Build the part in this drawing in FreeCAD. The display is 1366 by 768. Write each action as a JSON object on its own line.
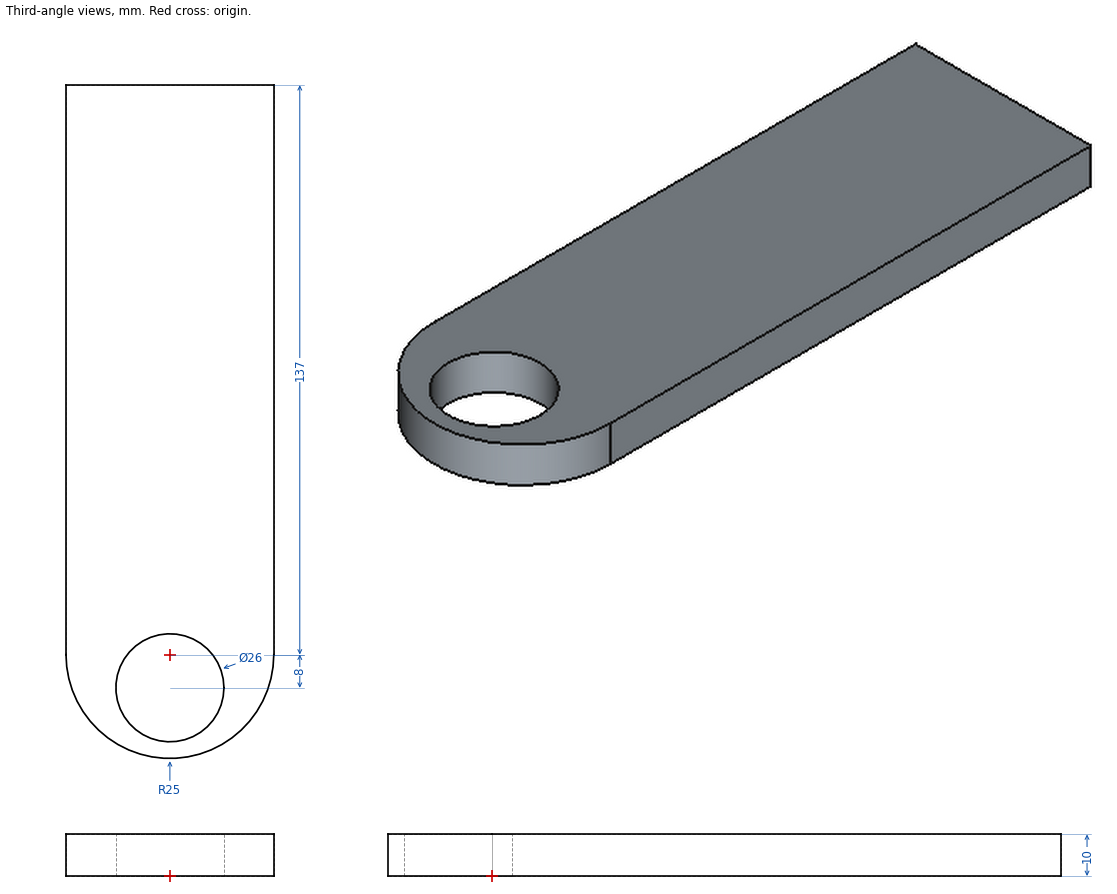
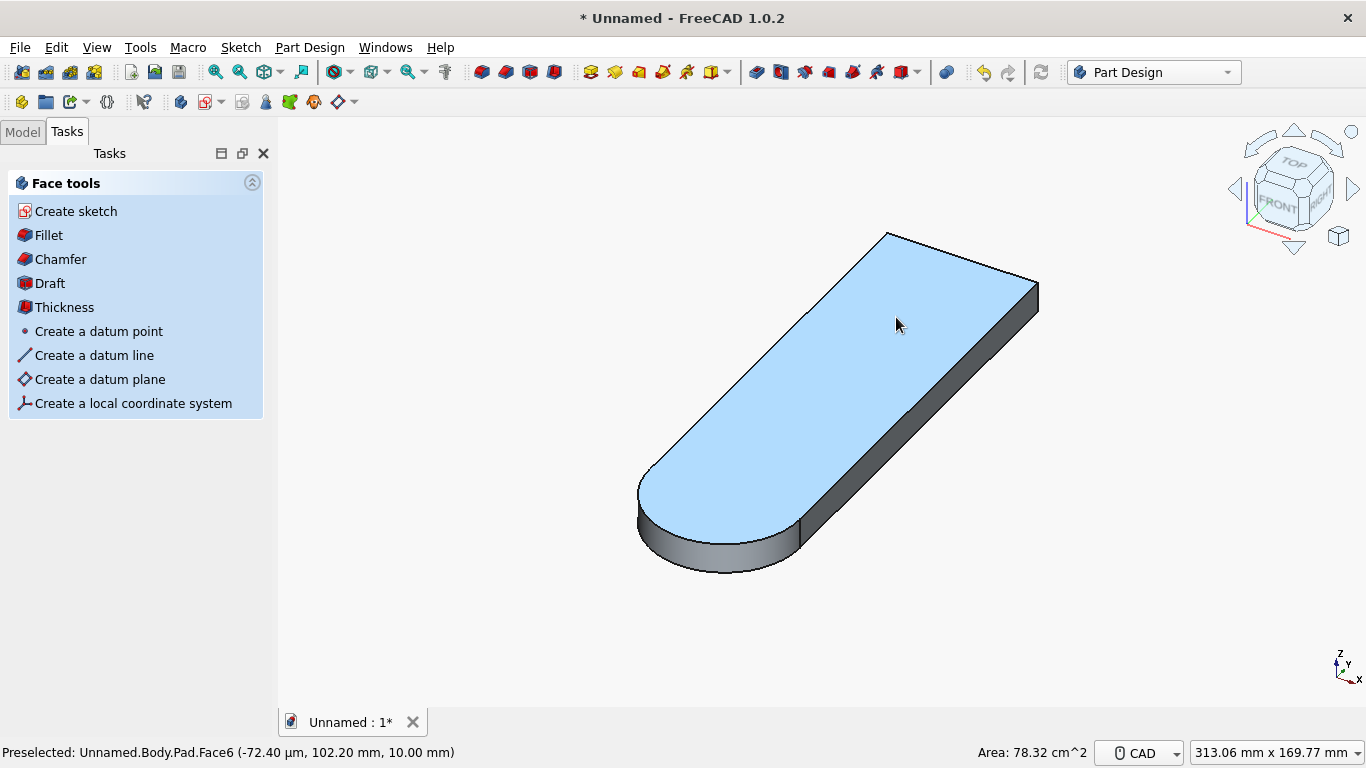
{"action": "left_click", "coordinate": [206, 102]}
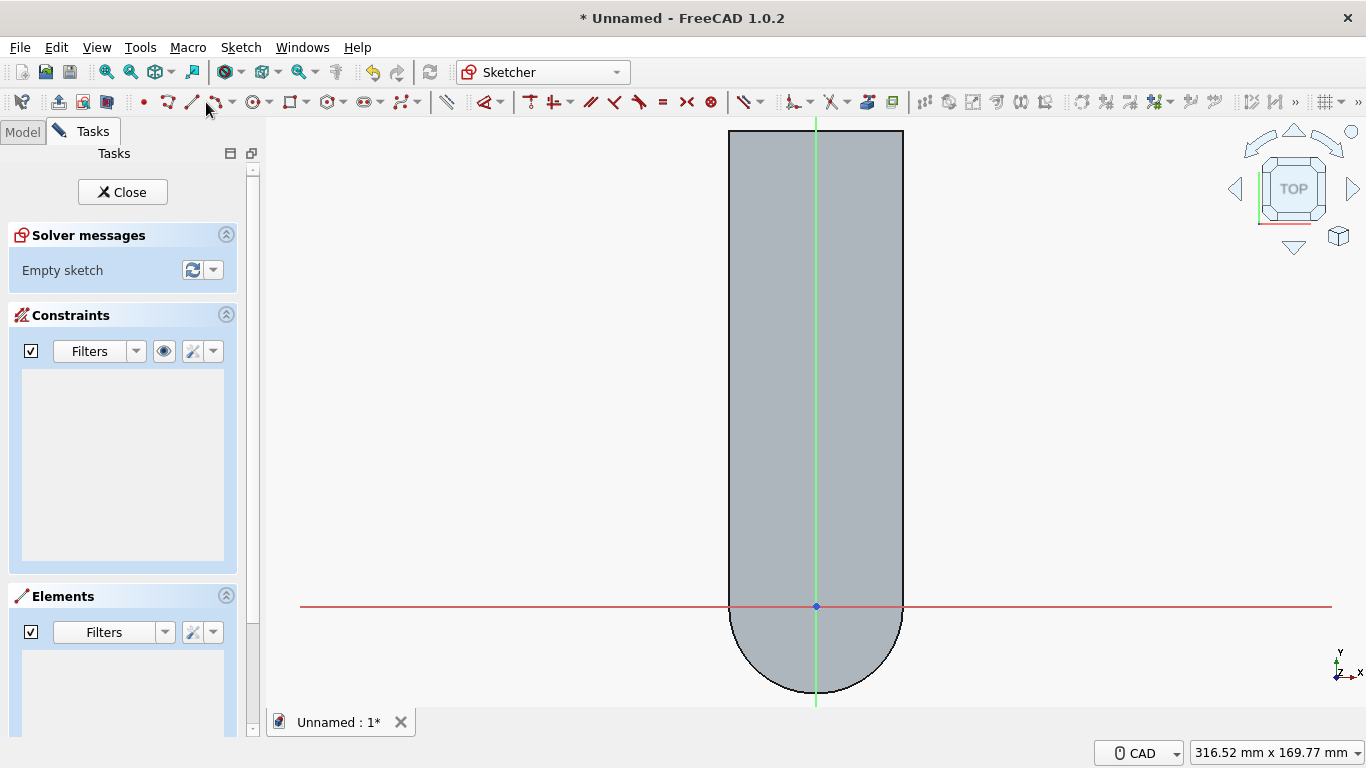
{"action": "scroll", "coordinate": [748, 412], "scroll_direction": "down", "scroll_amount": 5}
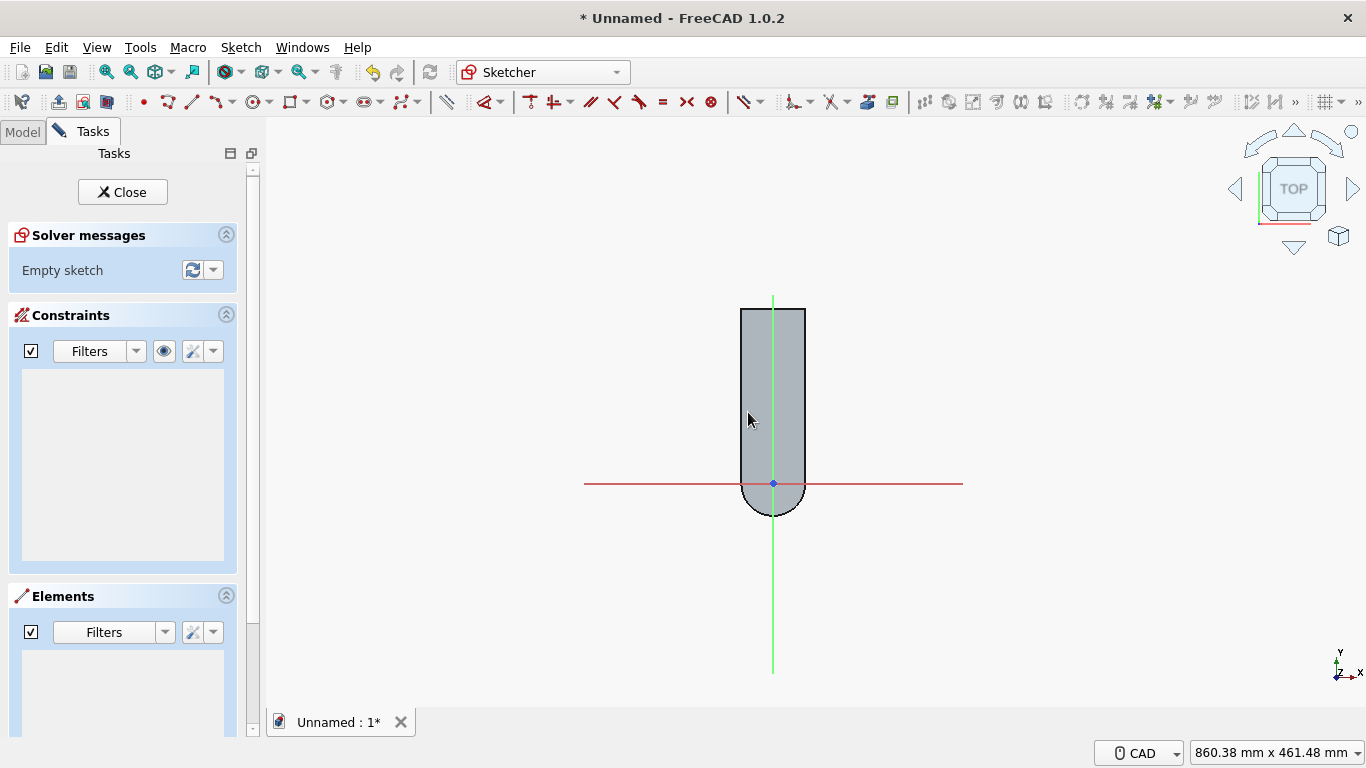
{"action": "scroll", "coordinate": [776, 502], "scroll_direction": "up", "scroll_amount": 12}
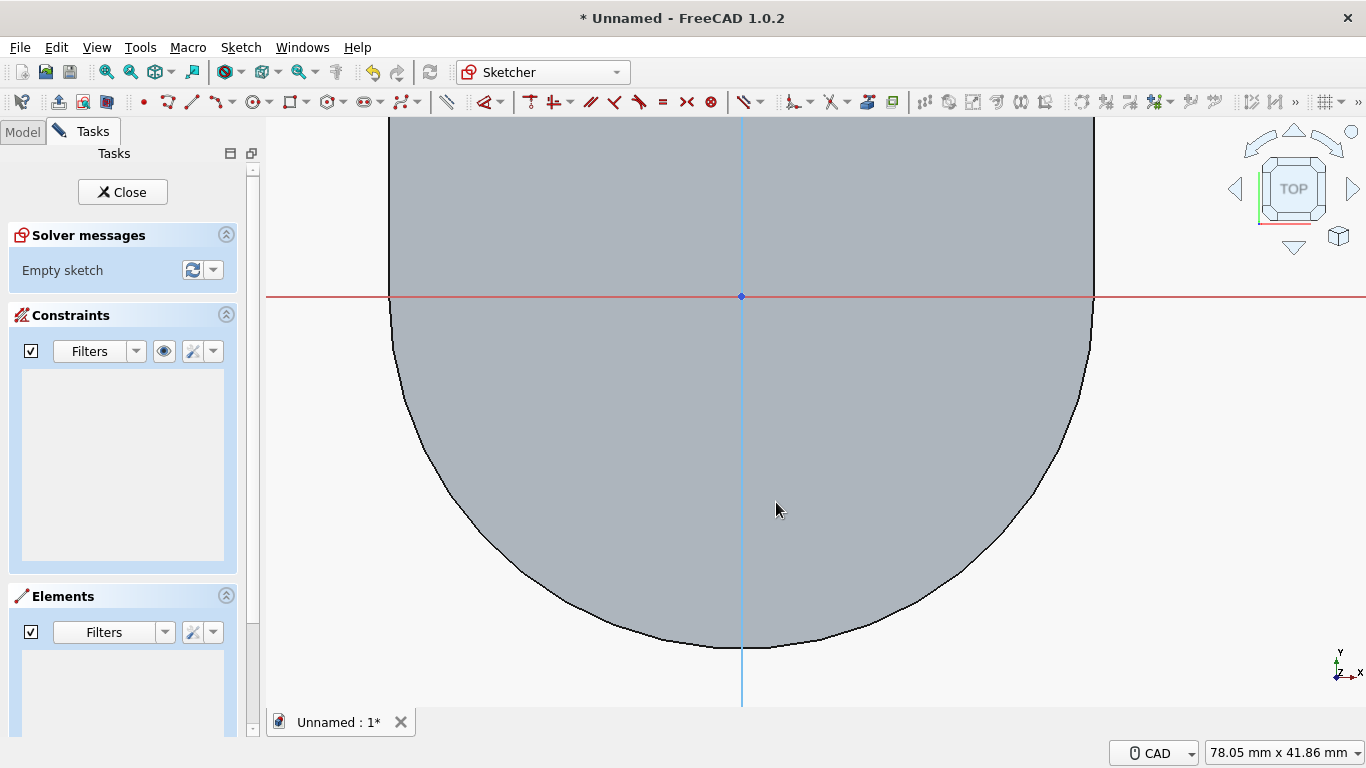
{"action": "left_click", "coordinate": [254, 102]}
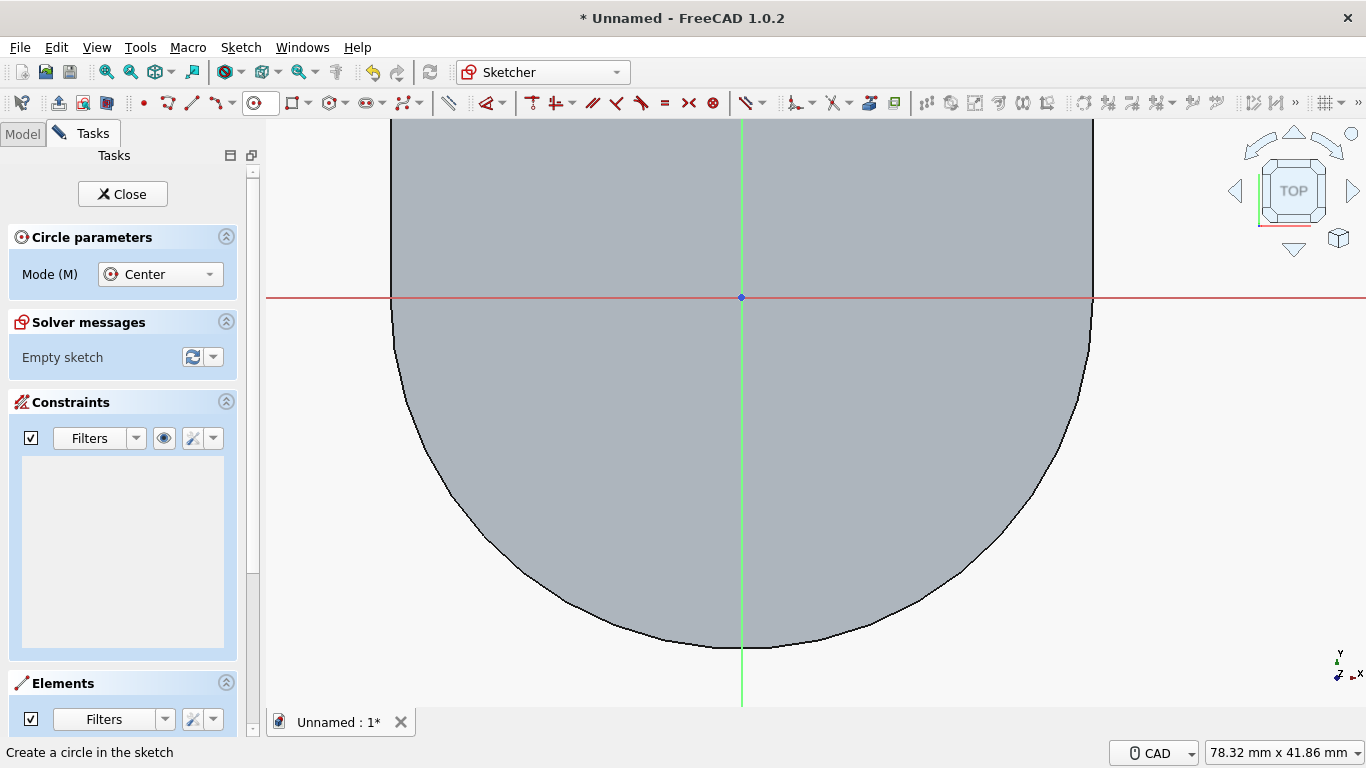
{"action": "left_click", "coordinate": [742, 410]}
{"action": "mouse_move", "coordinate": [871, 281]}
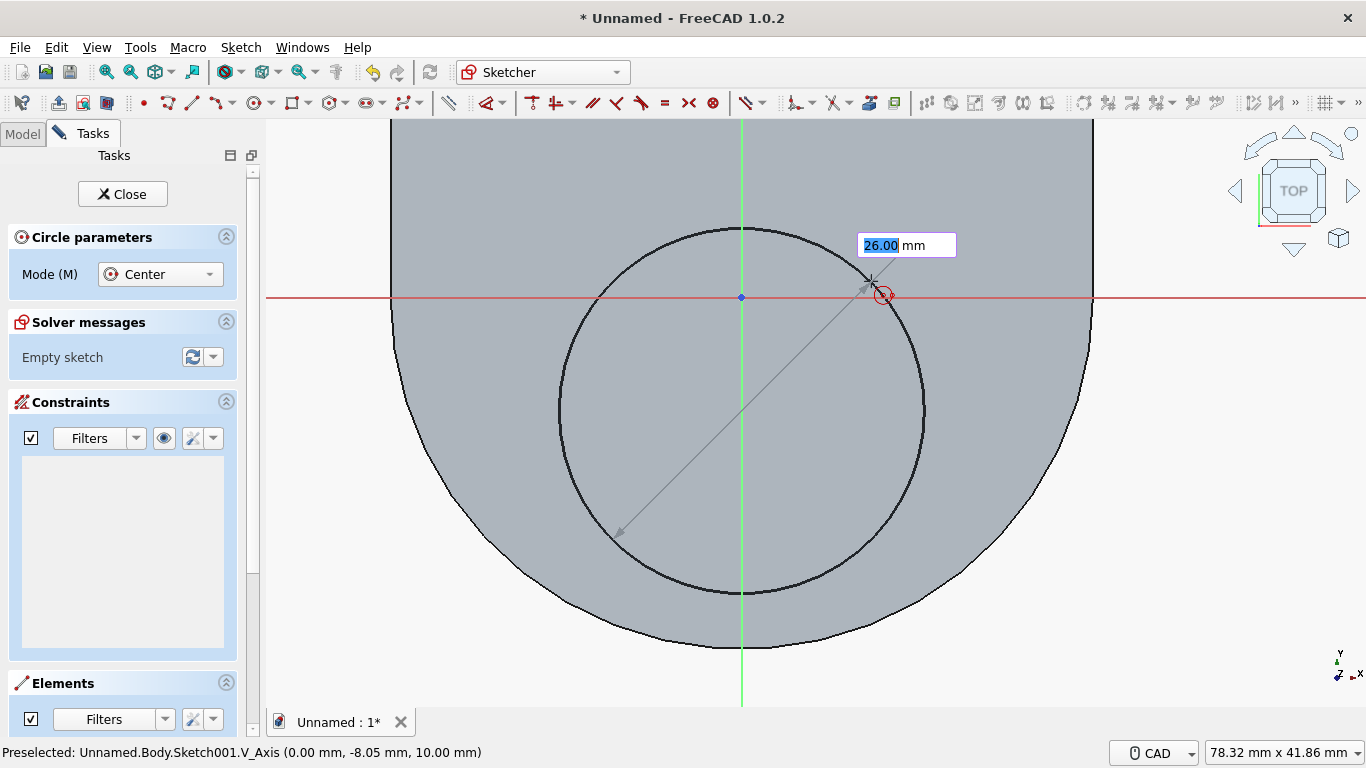
{"action": "type", "text": "26"}
{"action": "key", "text": "Return"}
{"action": "key", "text": "Escape"}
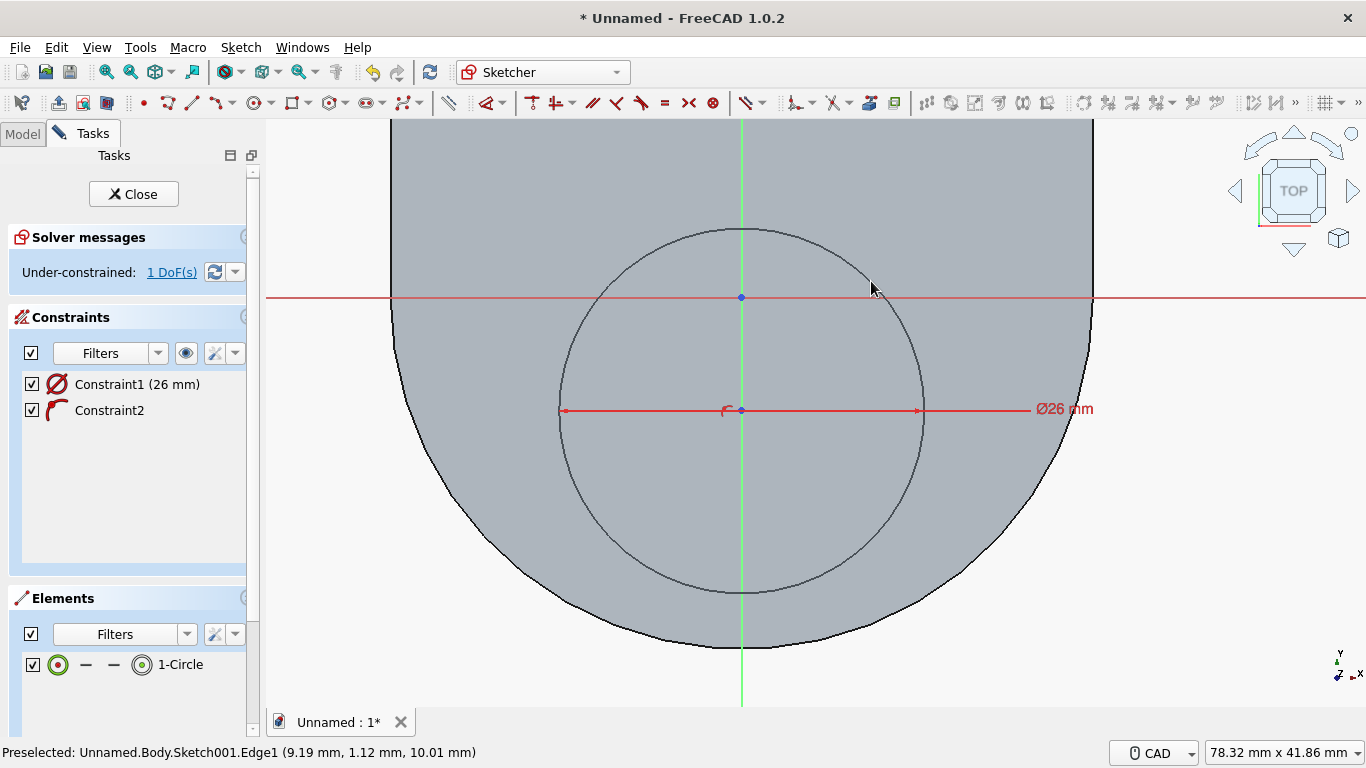
{"action": "left_click", "coordinate": [742, 411]}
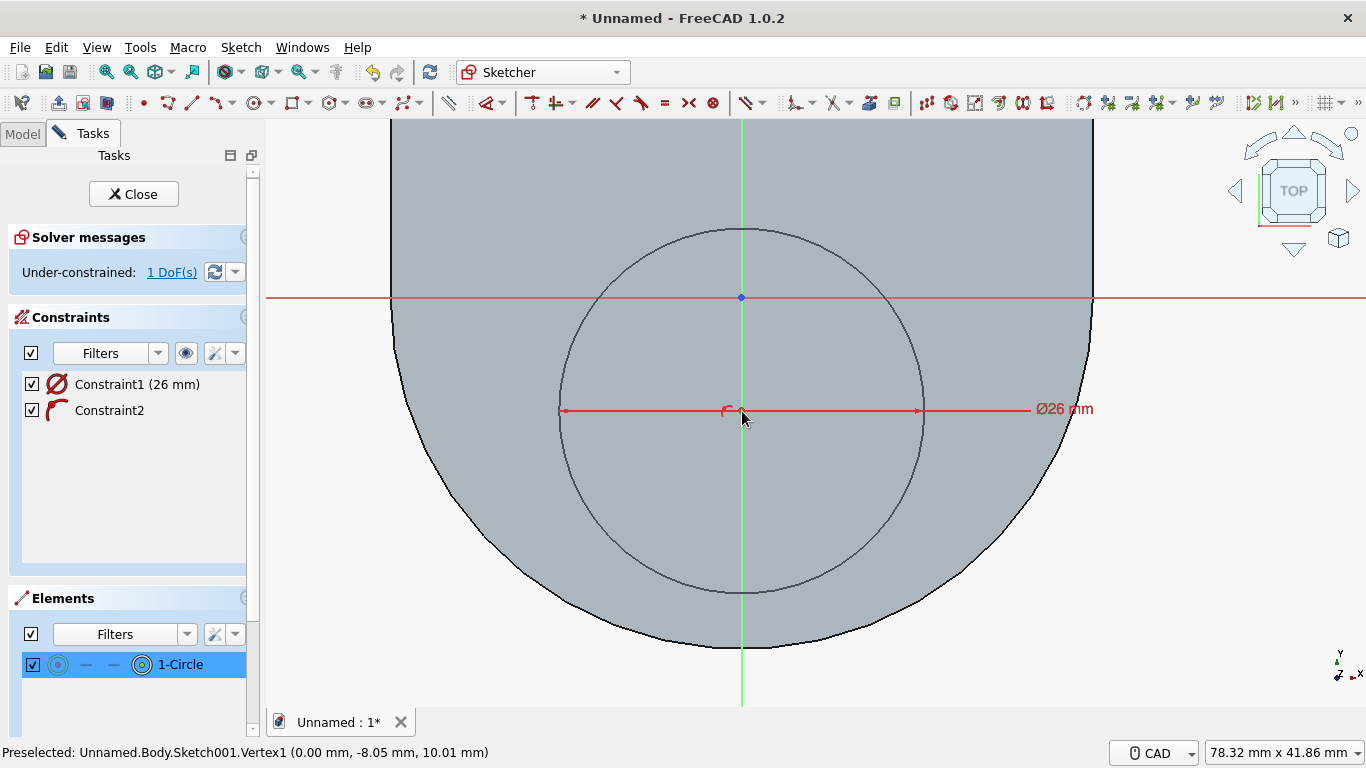
{"action": "key", "text": "i"}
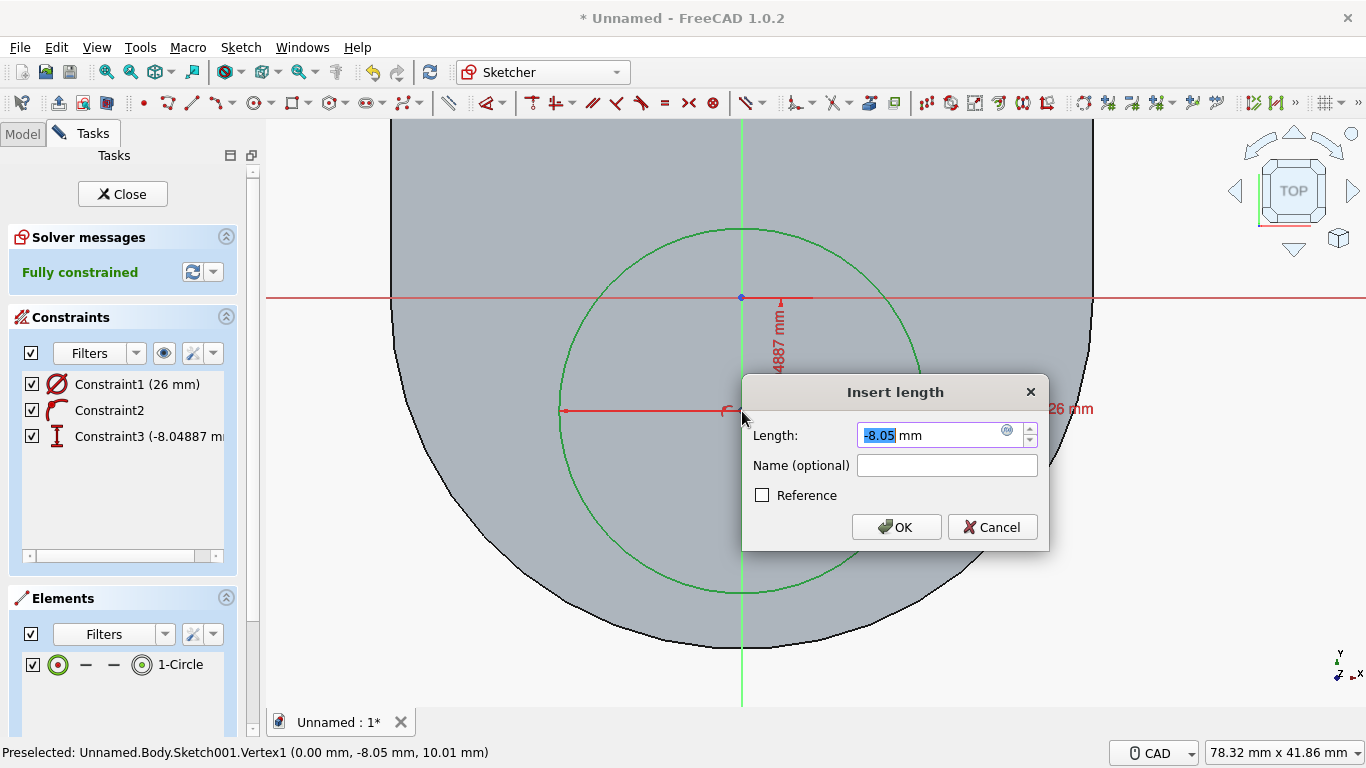
{"action": "type", "text": "-8"}
{"action": "key", "text": "Return"}